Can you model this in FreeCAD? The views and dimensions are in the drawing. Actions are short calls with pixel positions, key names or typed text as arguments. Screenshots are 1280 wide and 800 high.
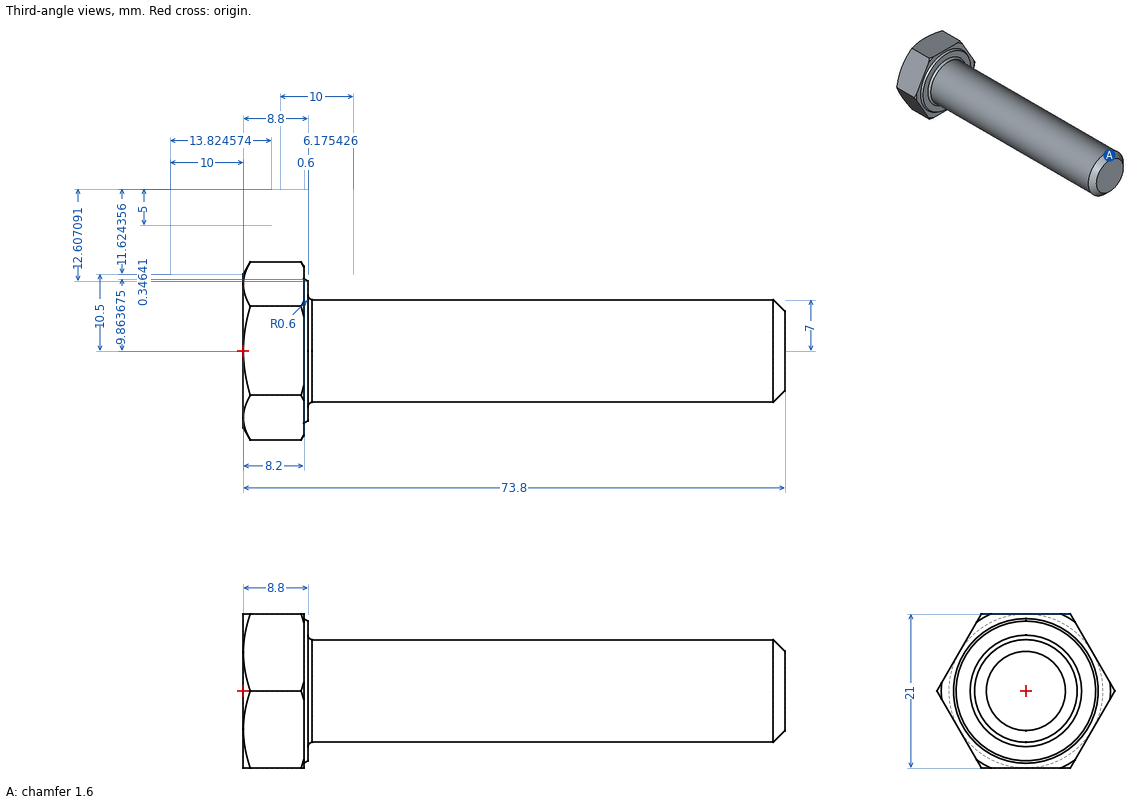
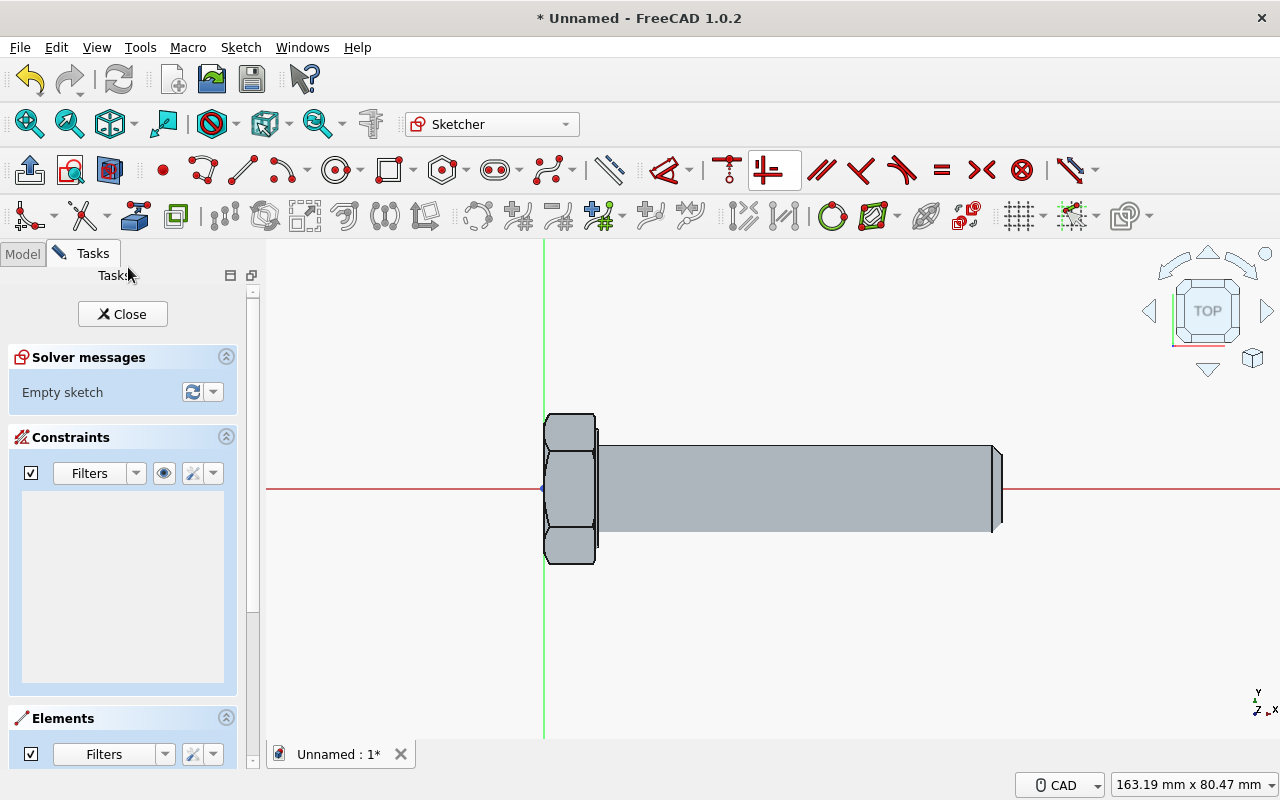
click(110, 170)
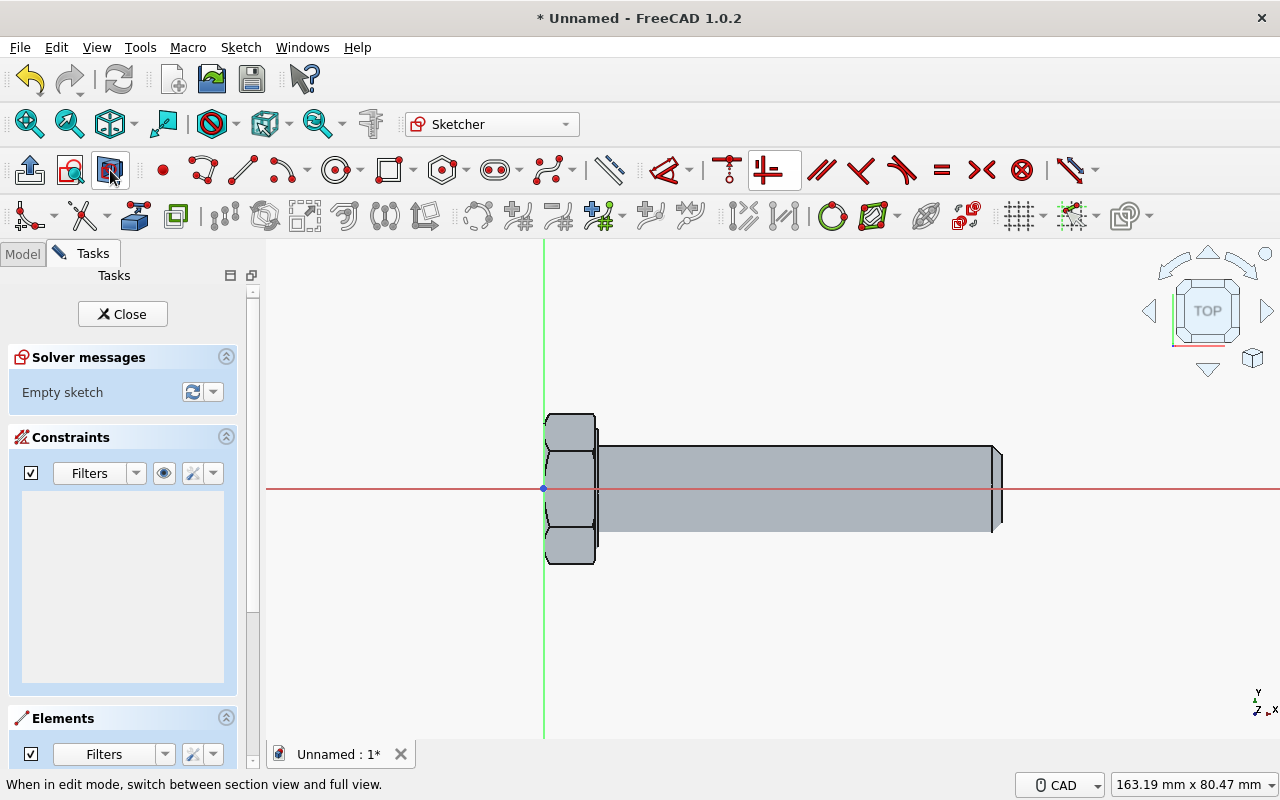
scroll(595, 441, up, 15)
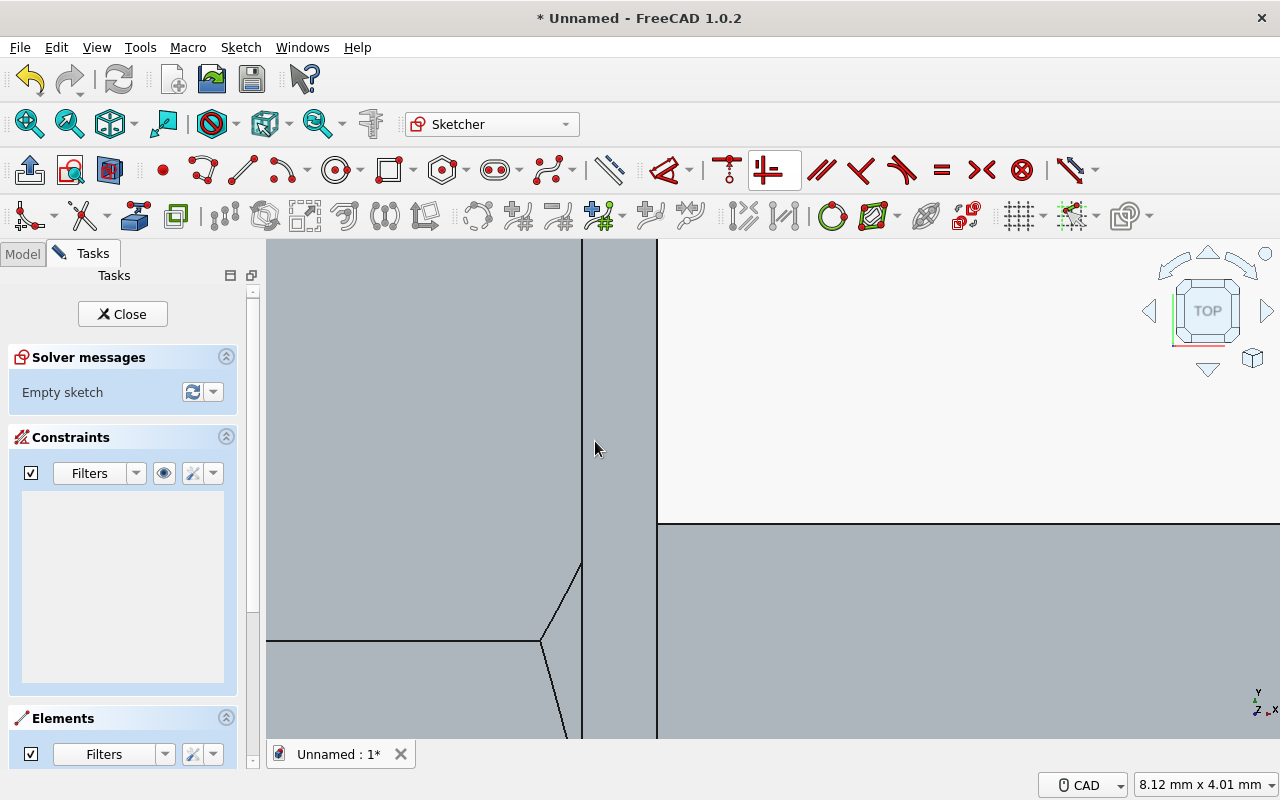
scroll(691, 485, up, 7)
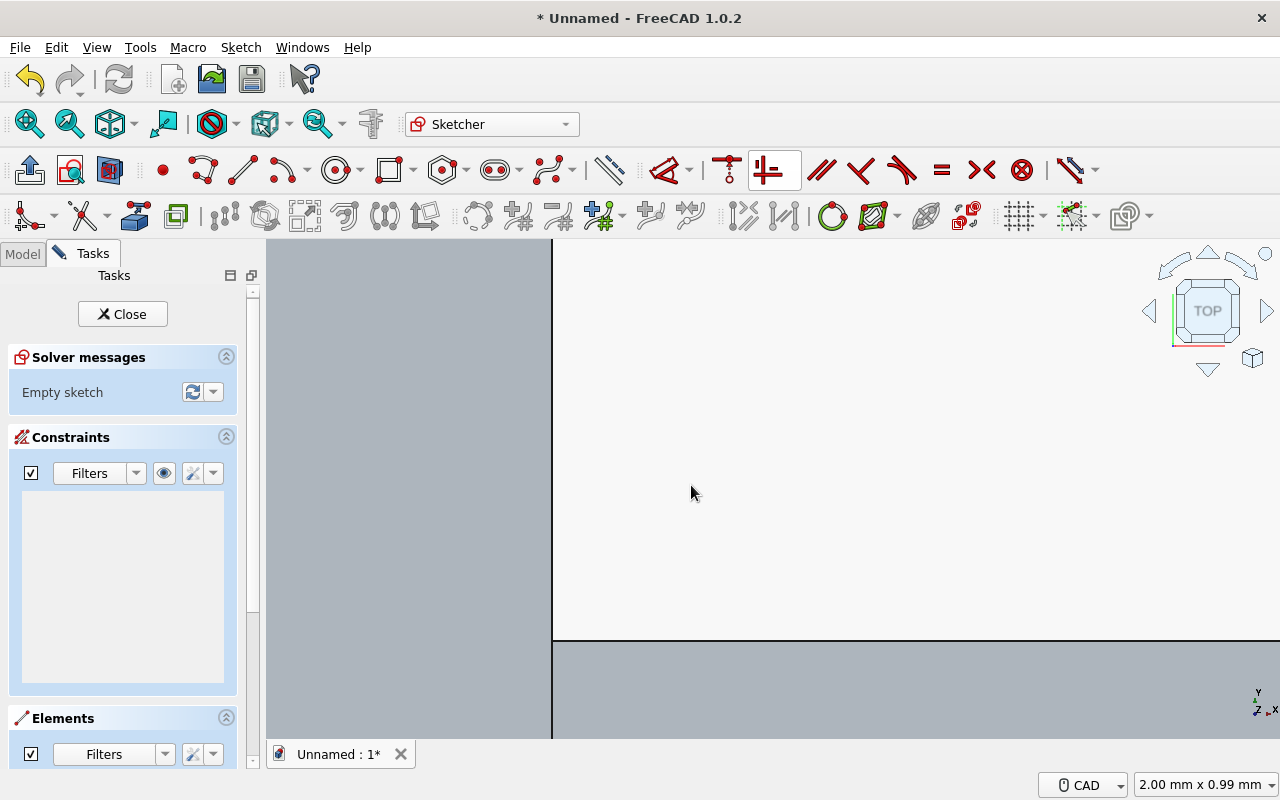
click(204, 170)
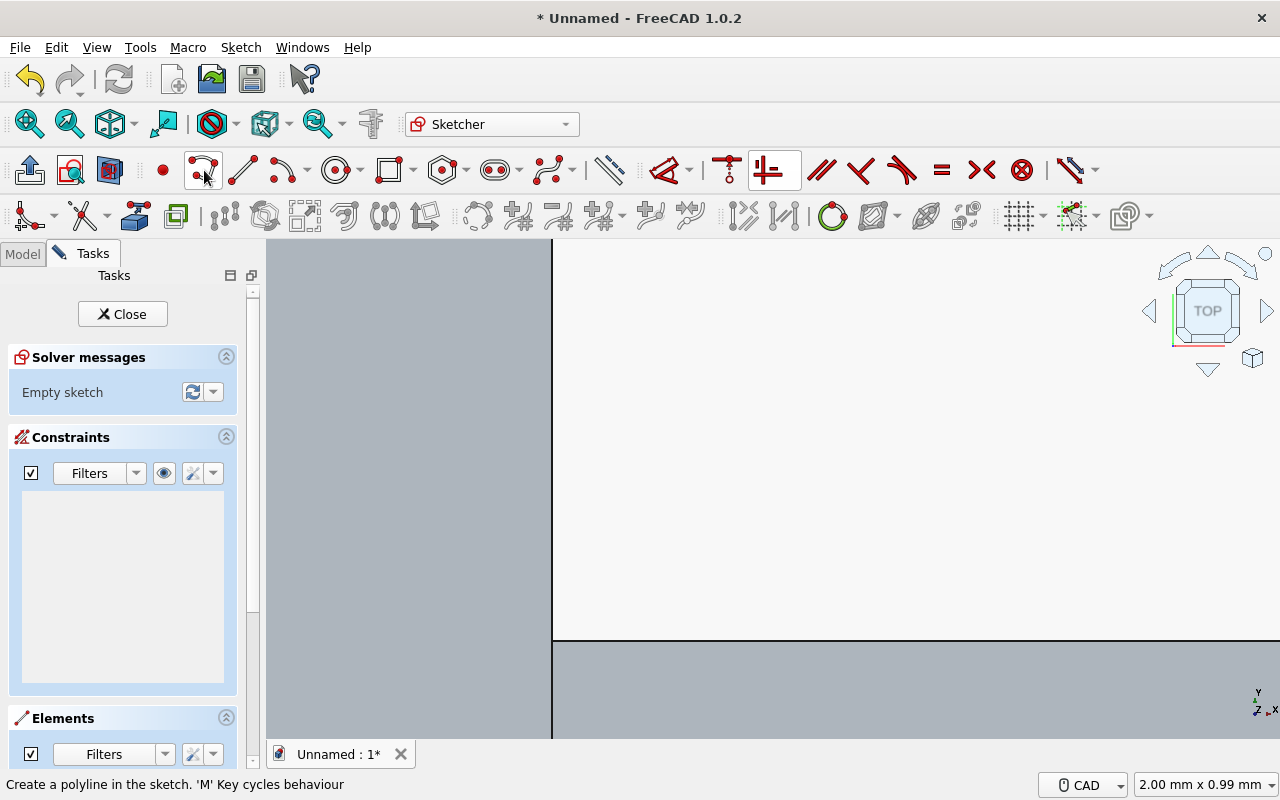
click(552, 337)
click(552, 641)
click(856, 641)
right_click(856, 641)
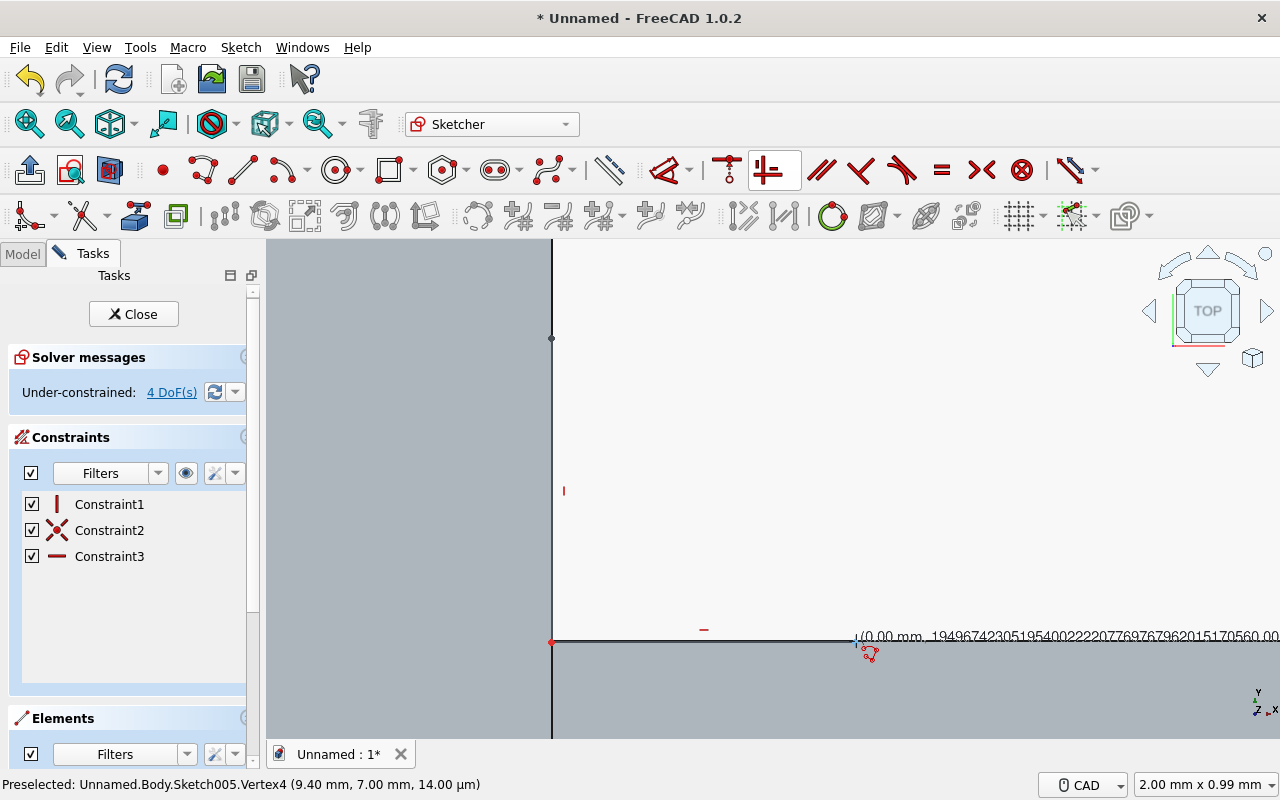
click(310, 170)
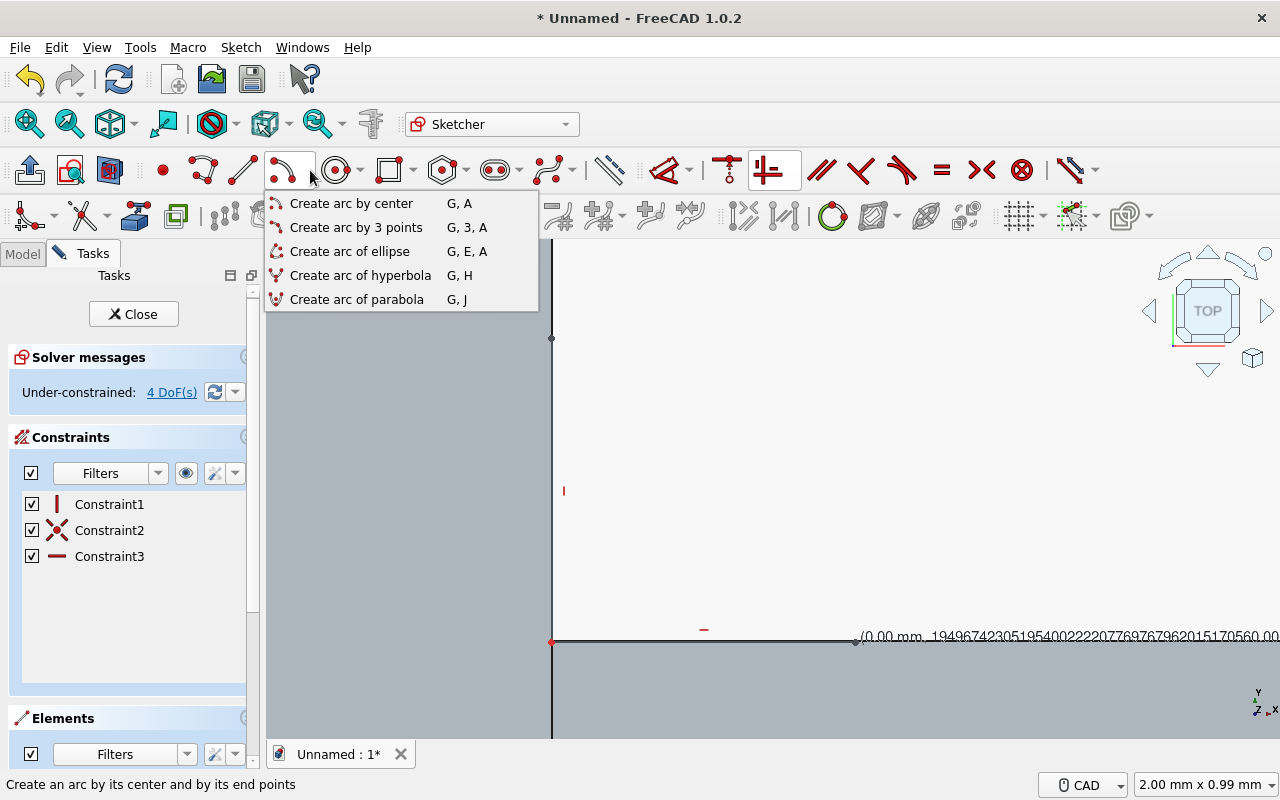
click(402, 227)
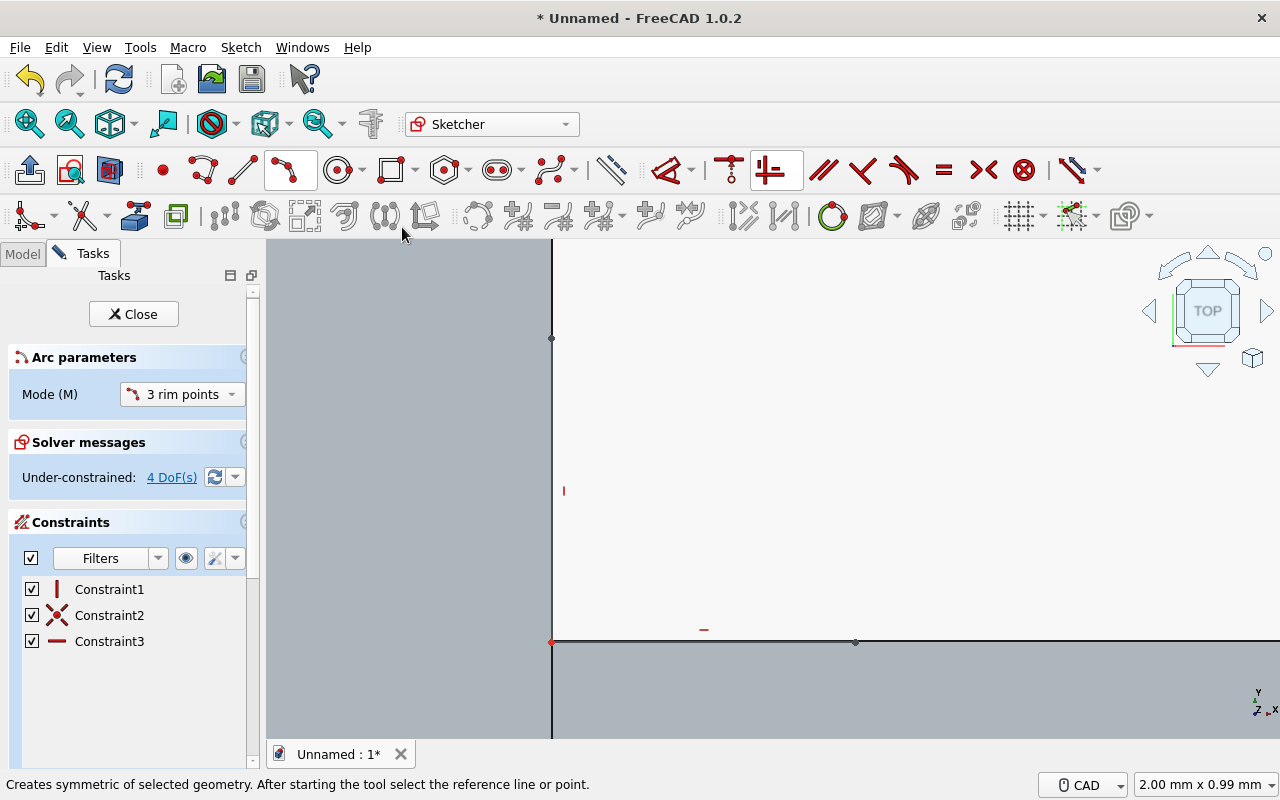
click(856, 642)
click(552, 338)
click(641, 552)
key(Escape)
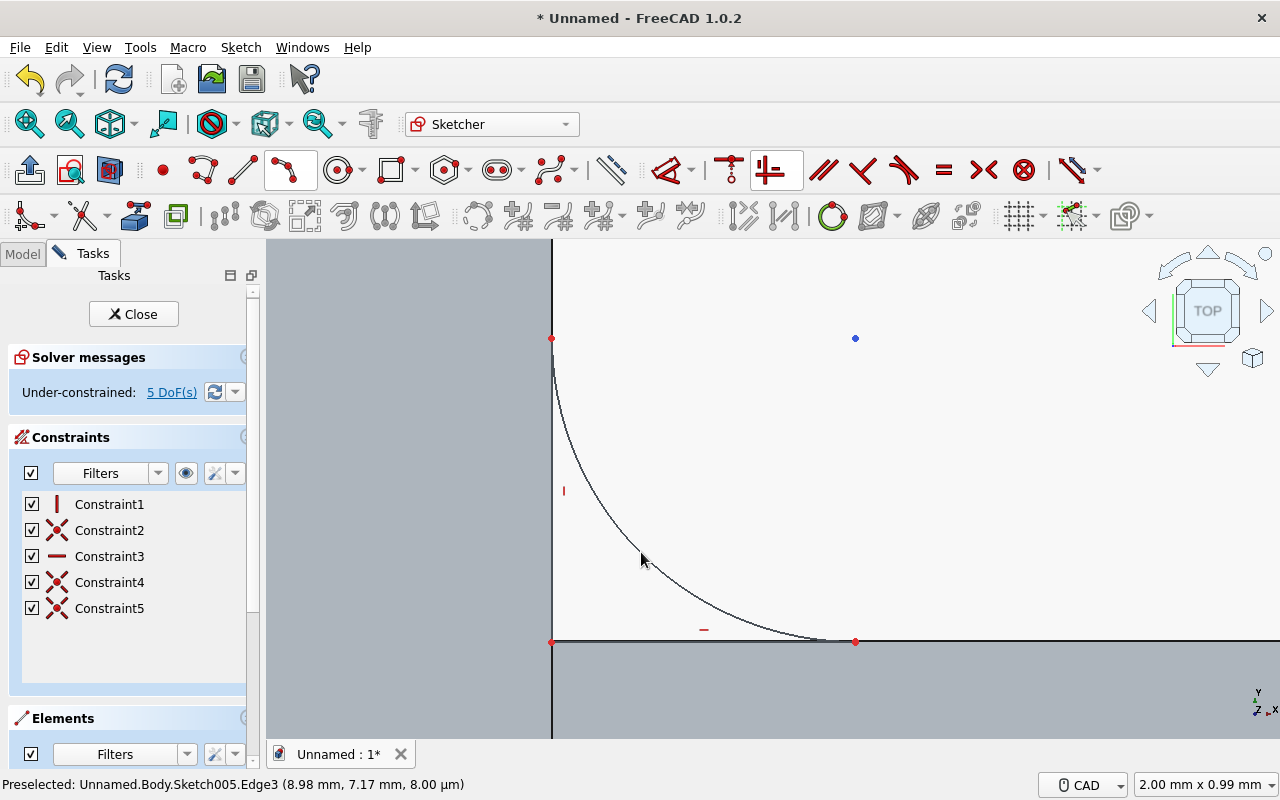
click(552, 429)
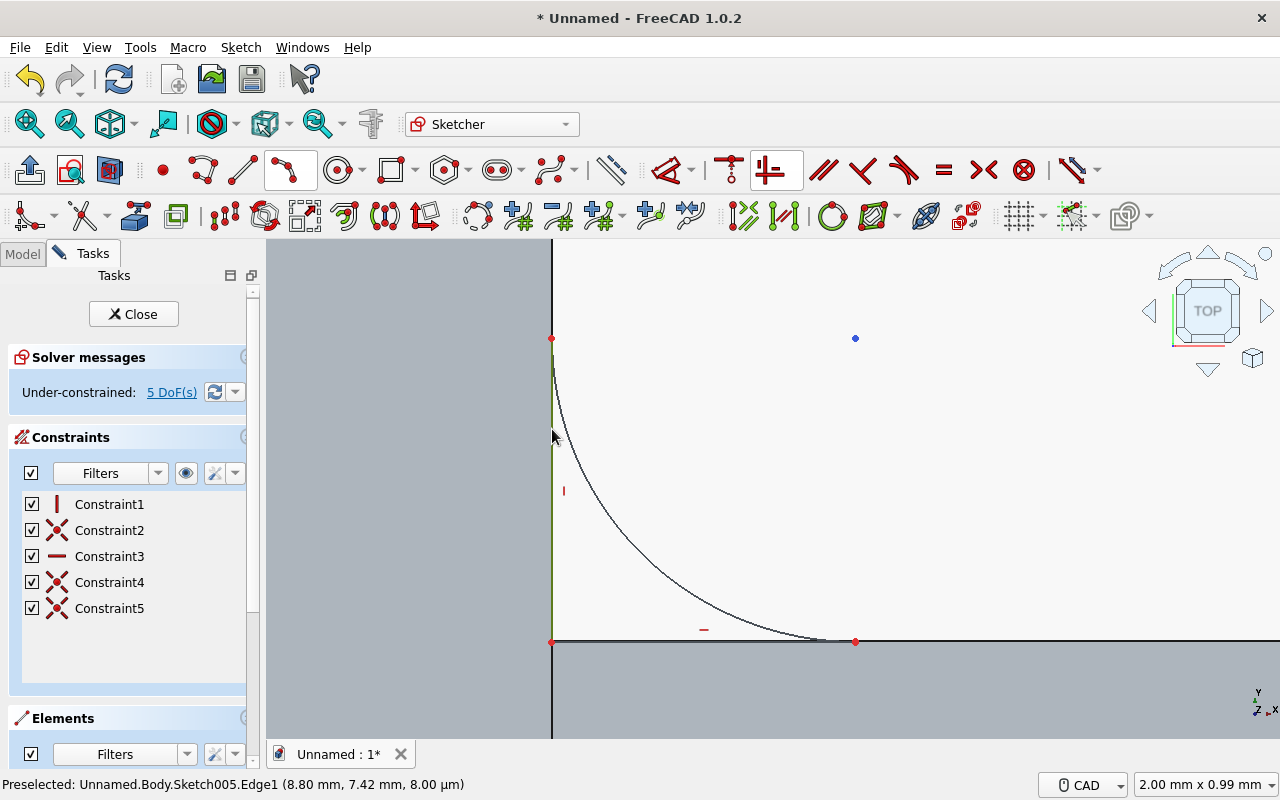
click(585, 476)